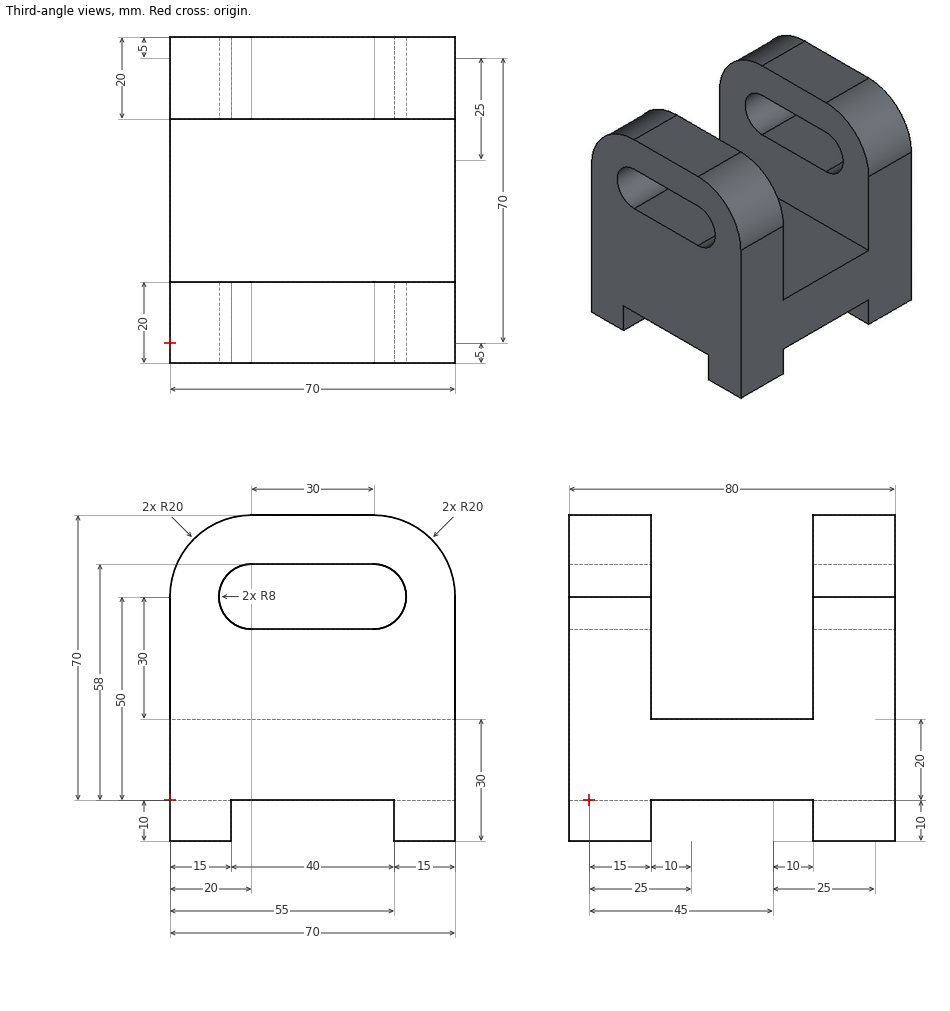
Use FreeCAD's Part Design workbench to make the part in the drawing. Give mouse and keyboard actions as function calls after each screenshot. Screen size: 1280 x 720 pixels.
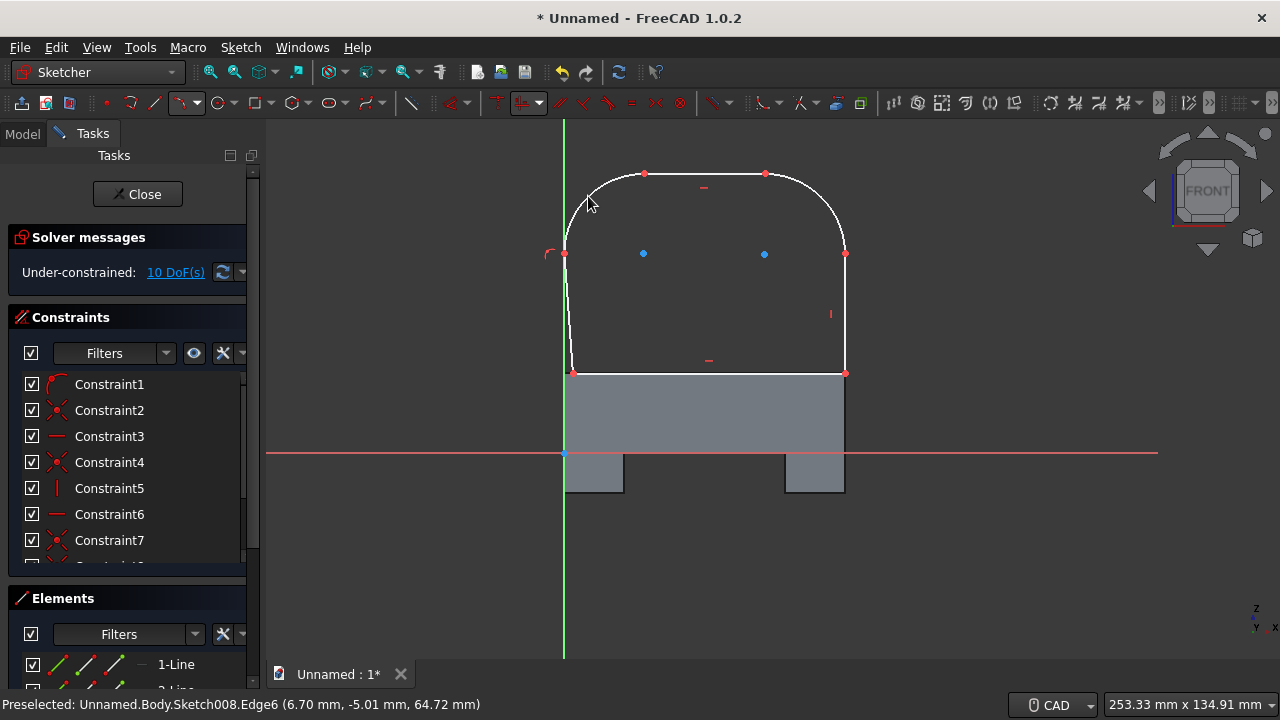
click(567, 290)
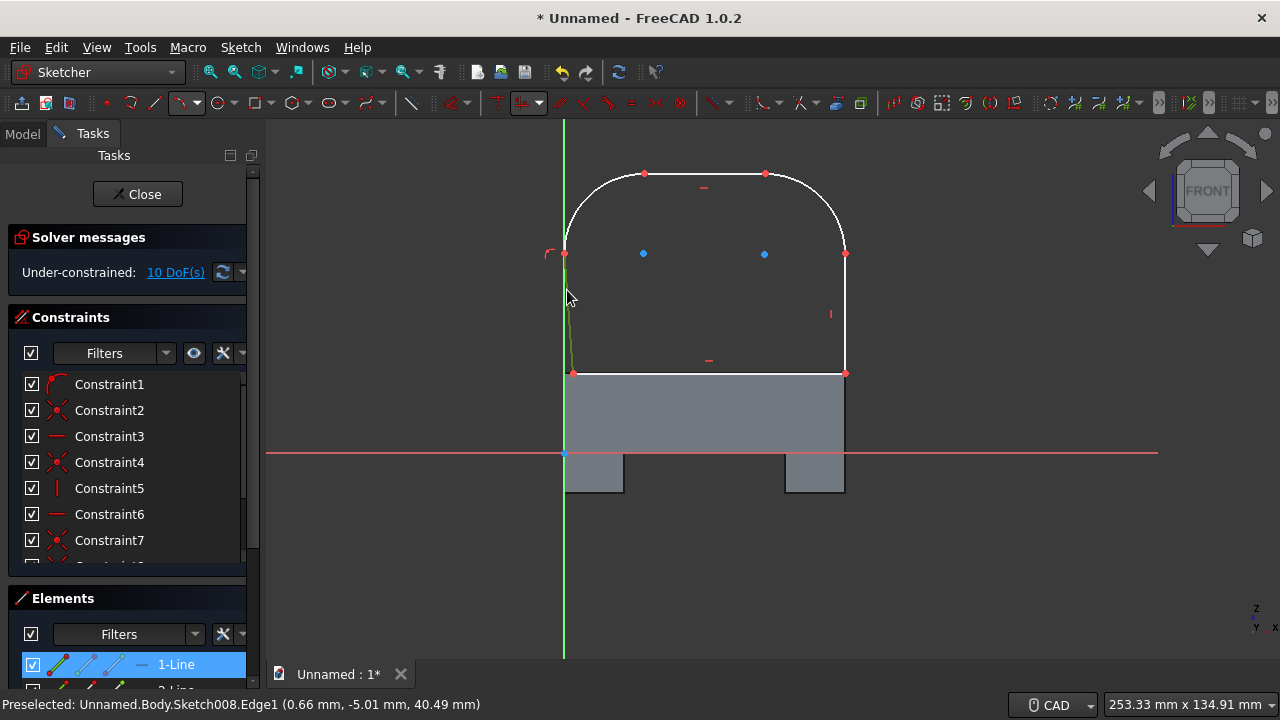
click(608, 183)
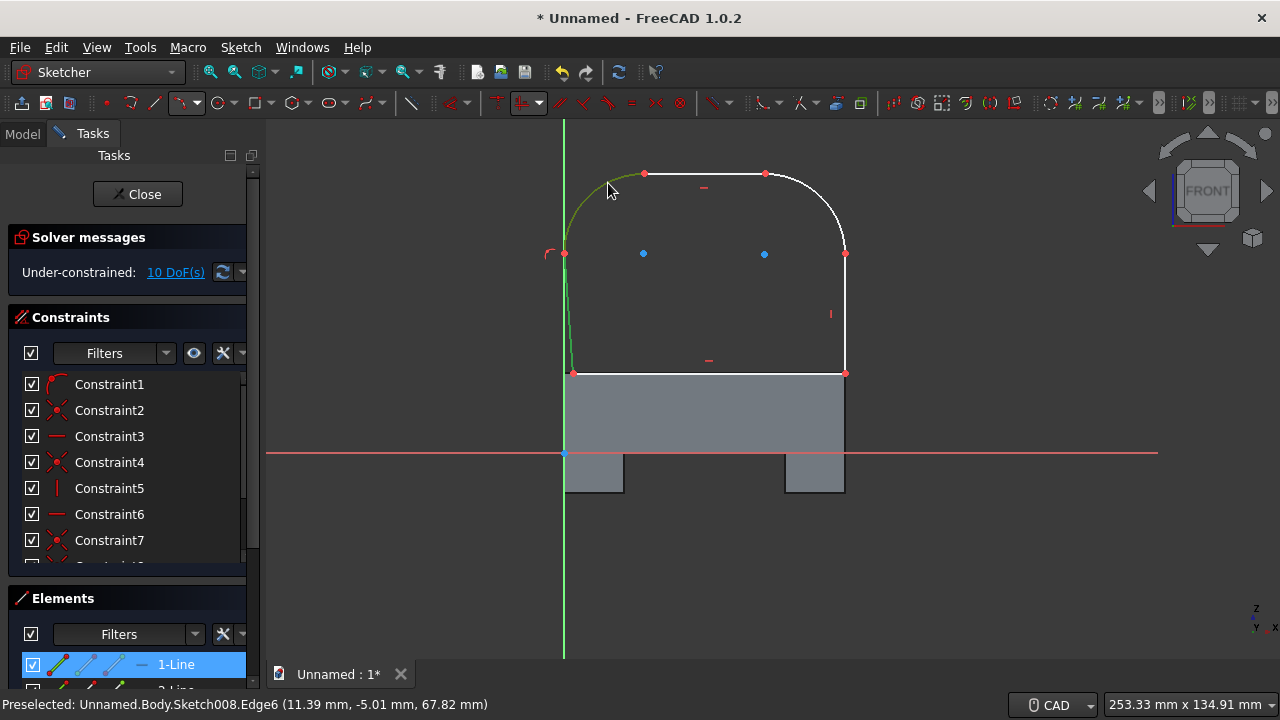
key(t)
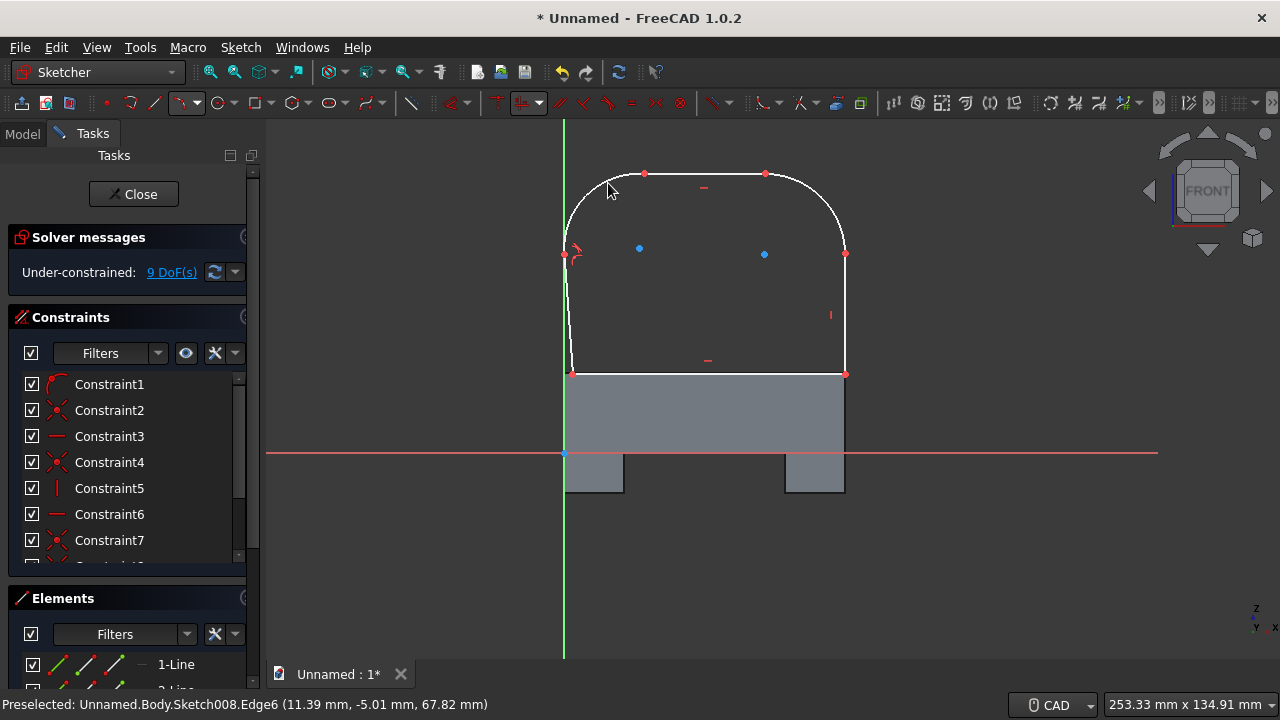
click(845, 338)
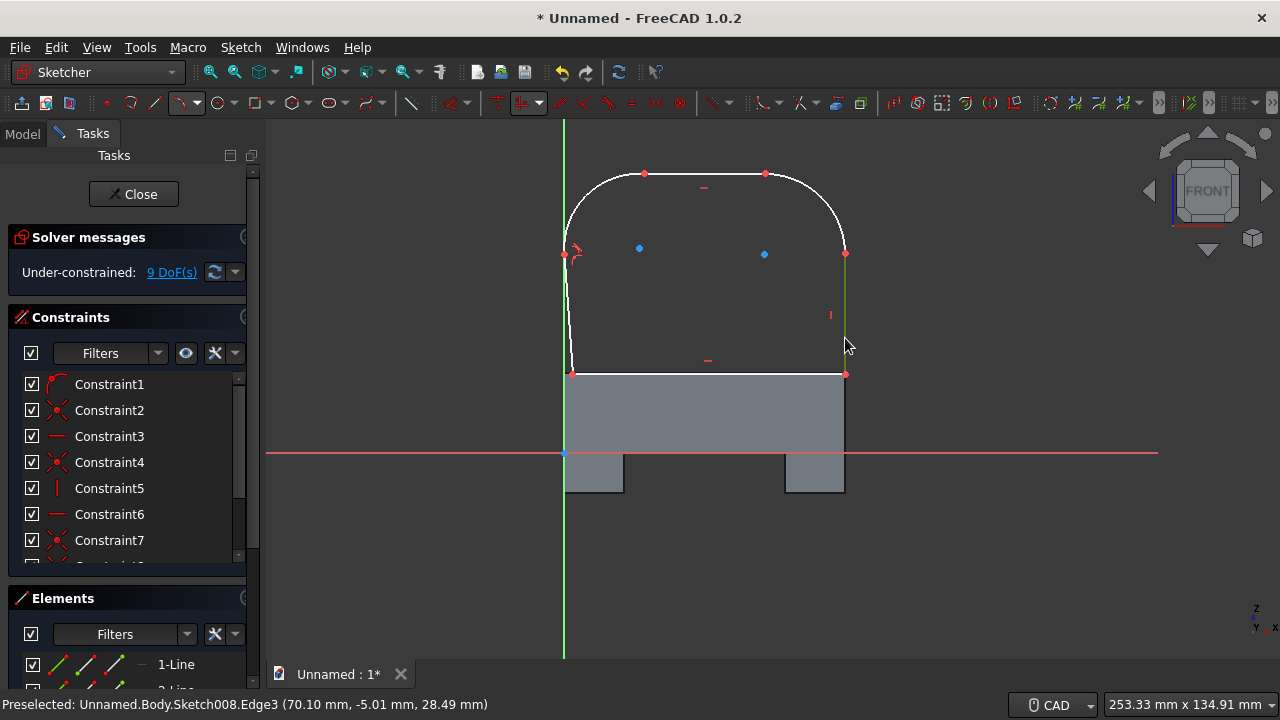
click(836, 218)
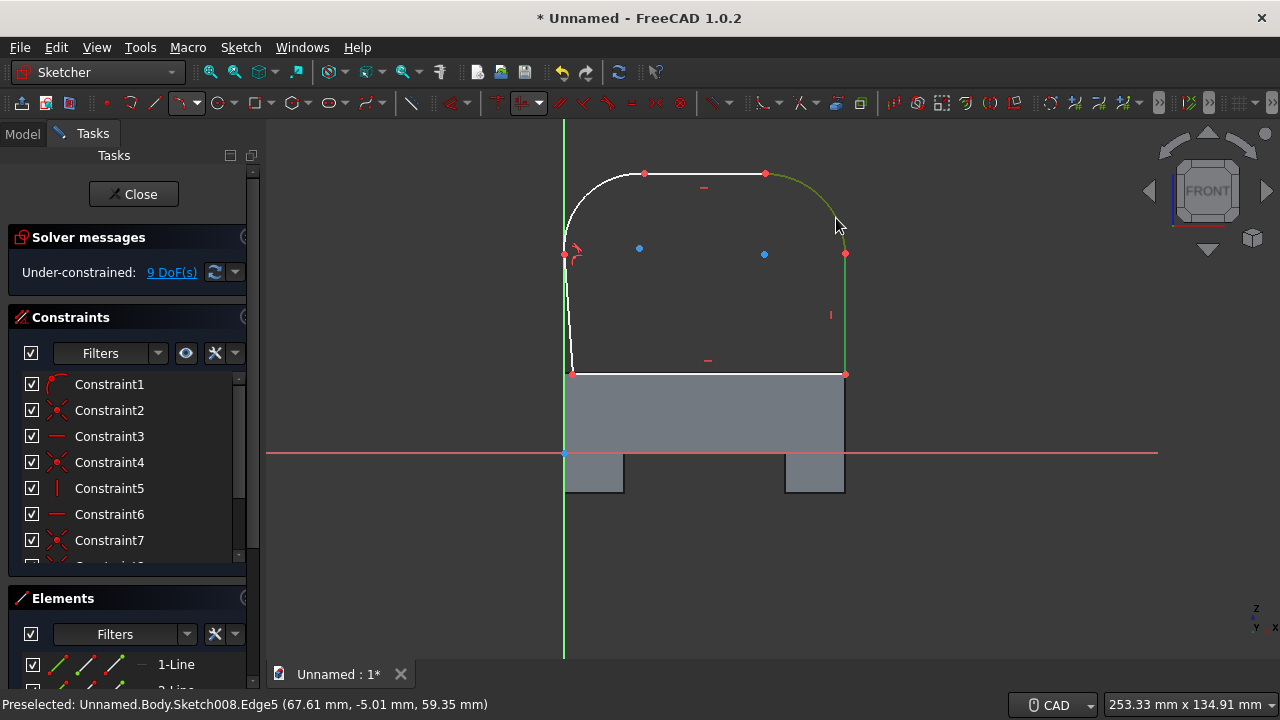
key(t)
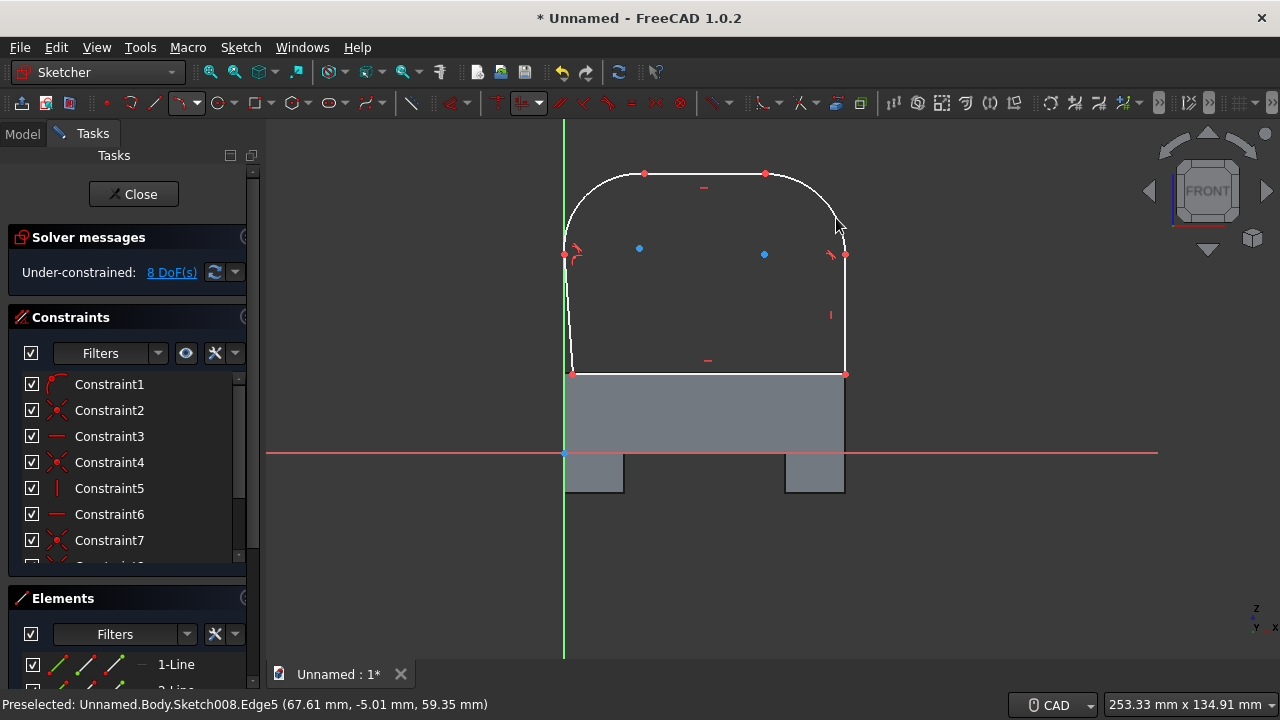
click(729, 174)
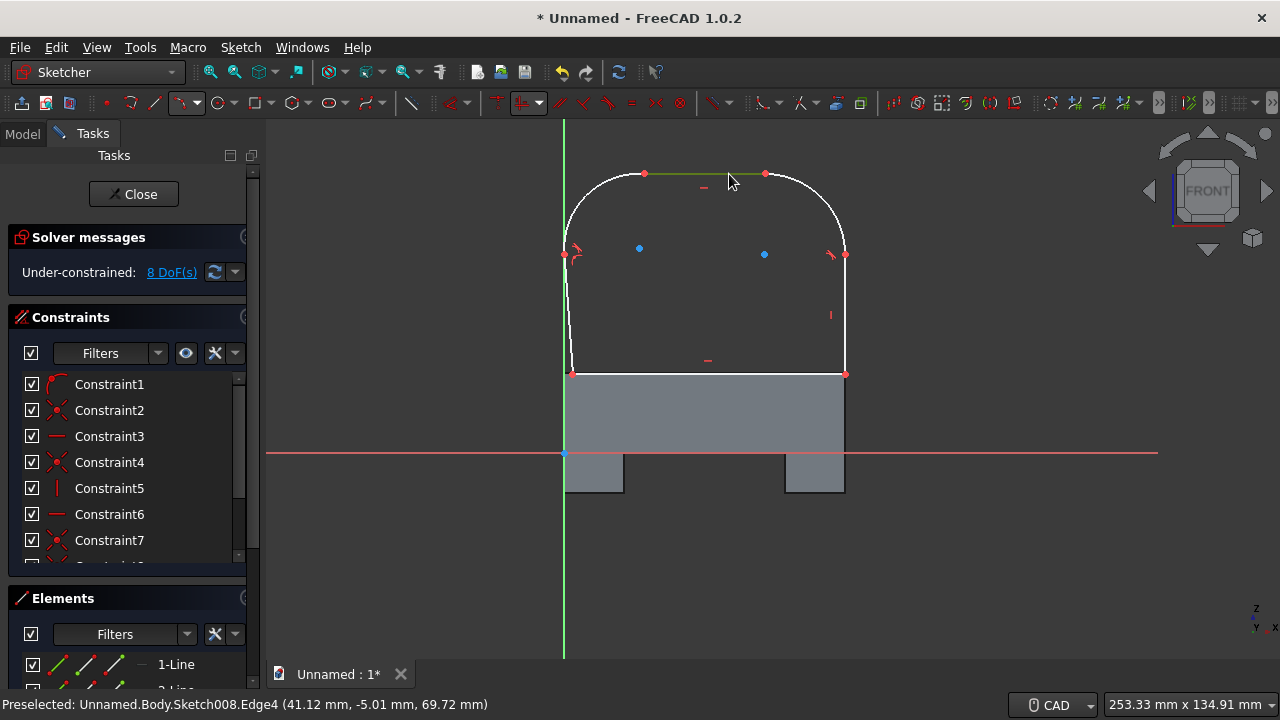
click(836, 218)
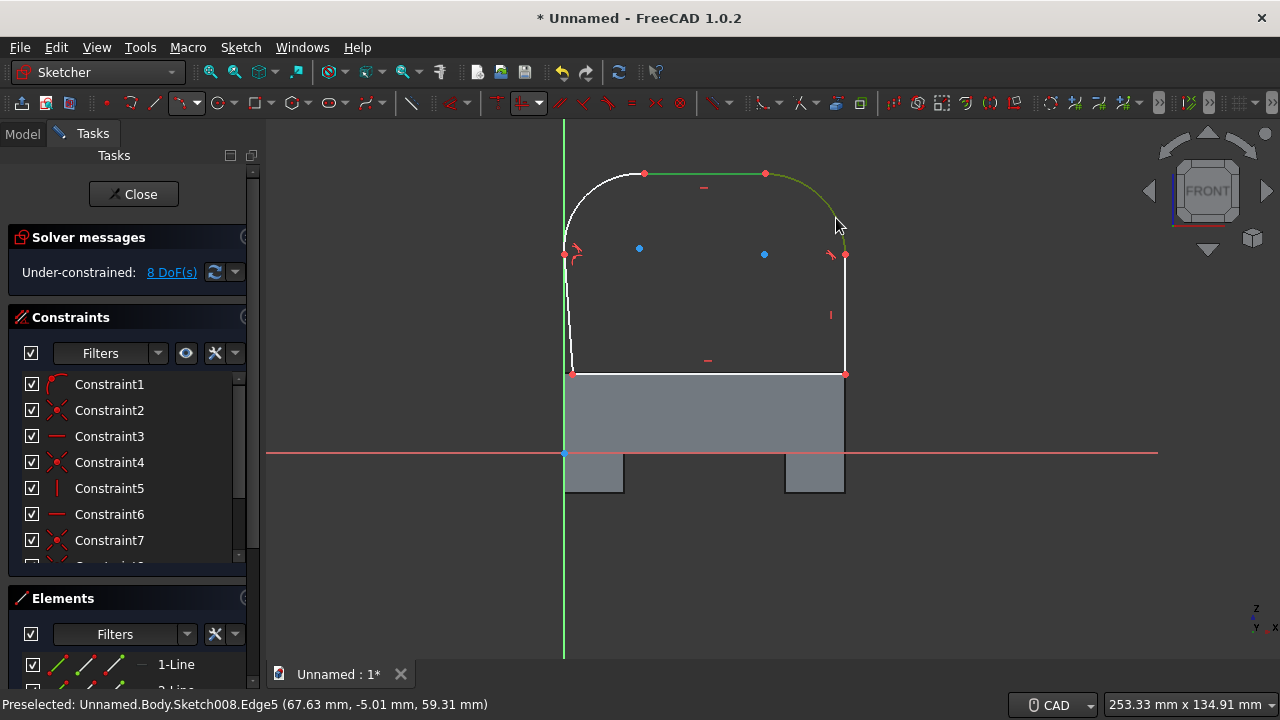
key(t)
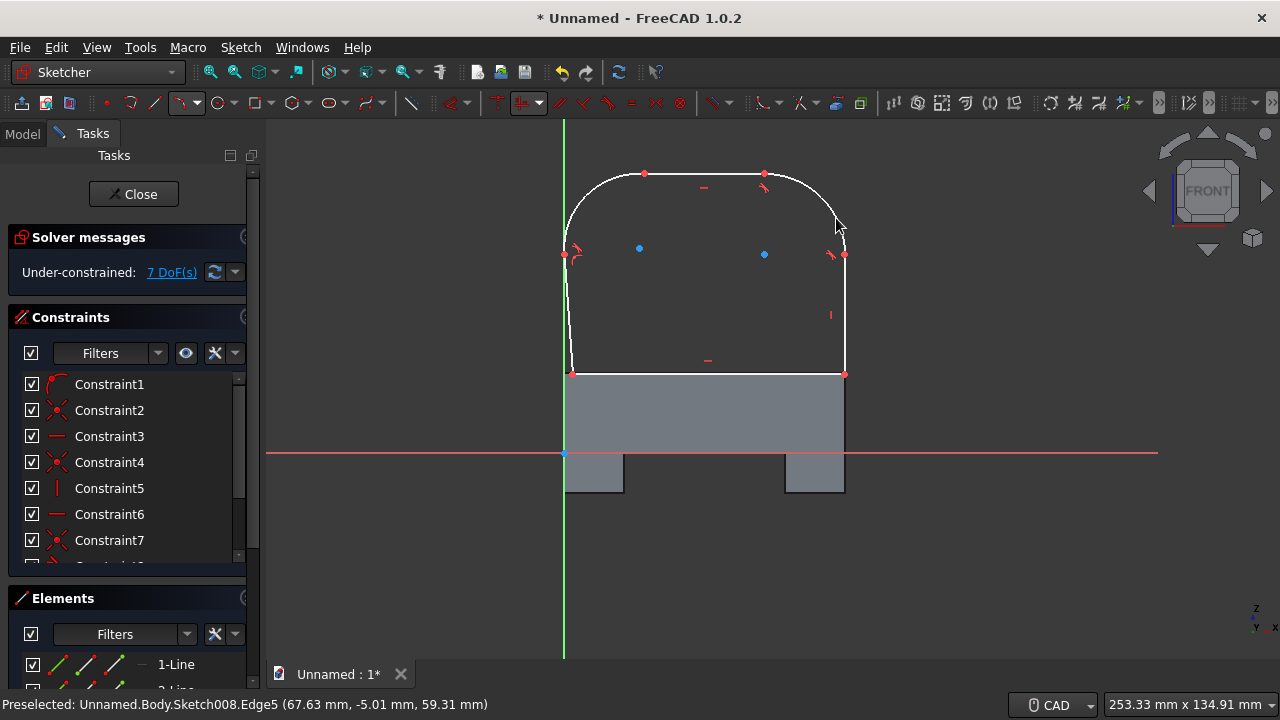
click(729, 174)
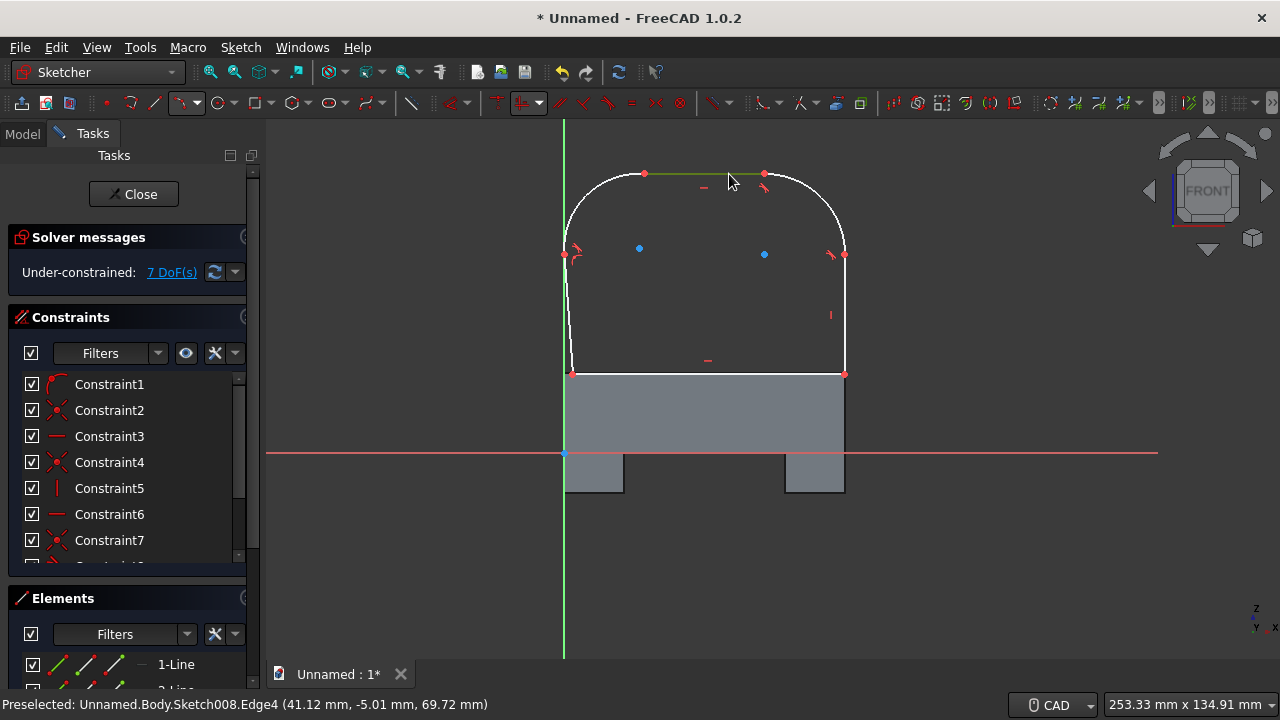
click(607, 181)